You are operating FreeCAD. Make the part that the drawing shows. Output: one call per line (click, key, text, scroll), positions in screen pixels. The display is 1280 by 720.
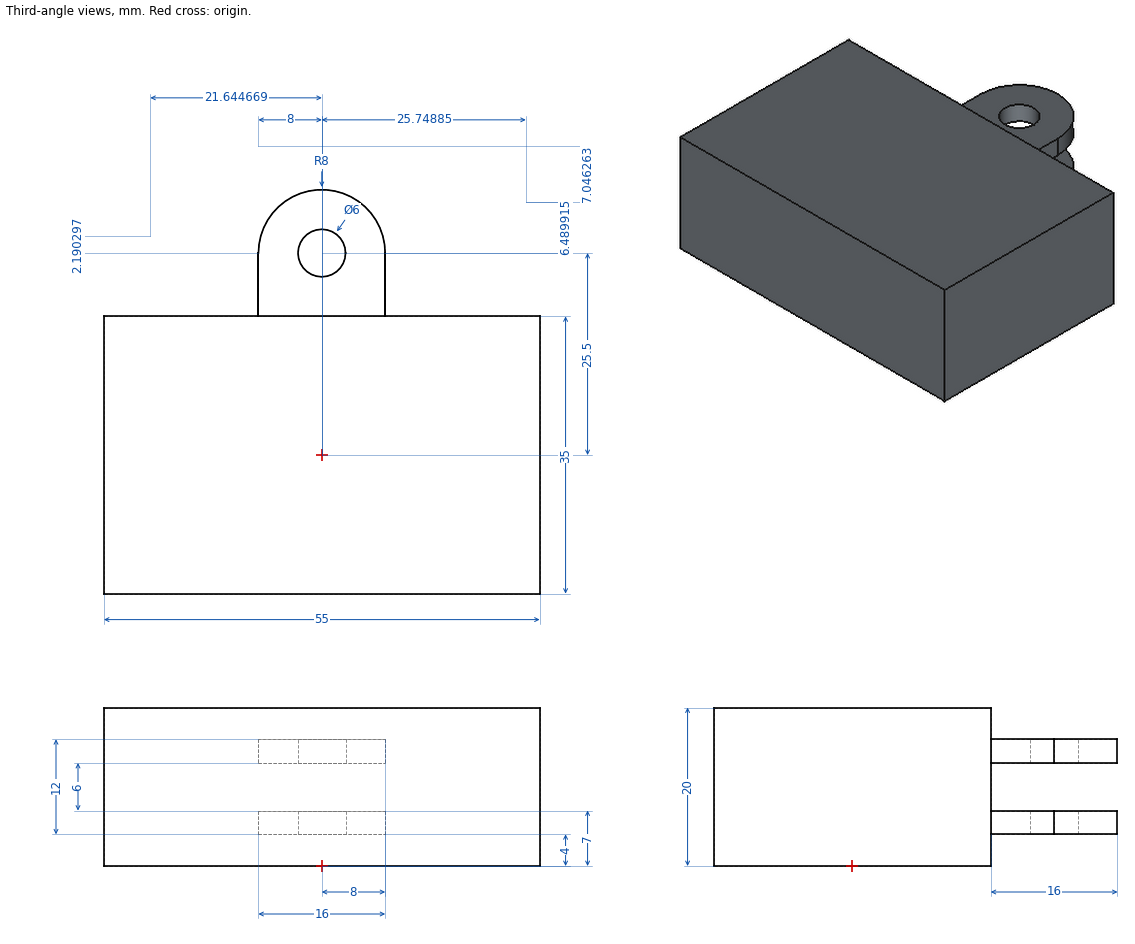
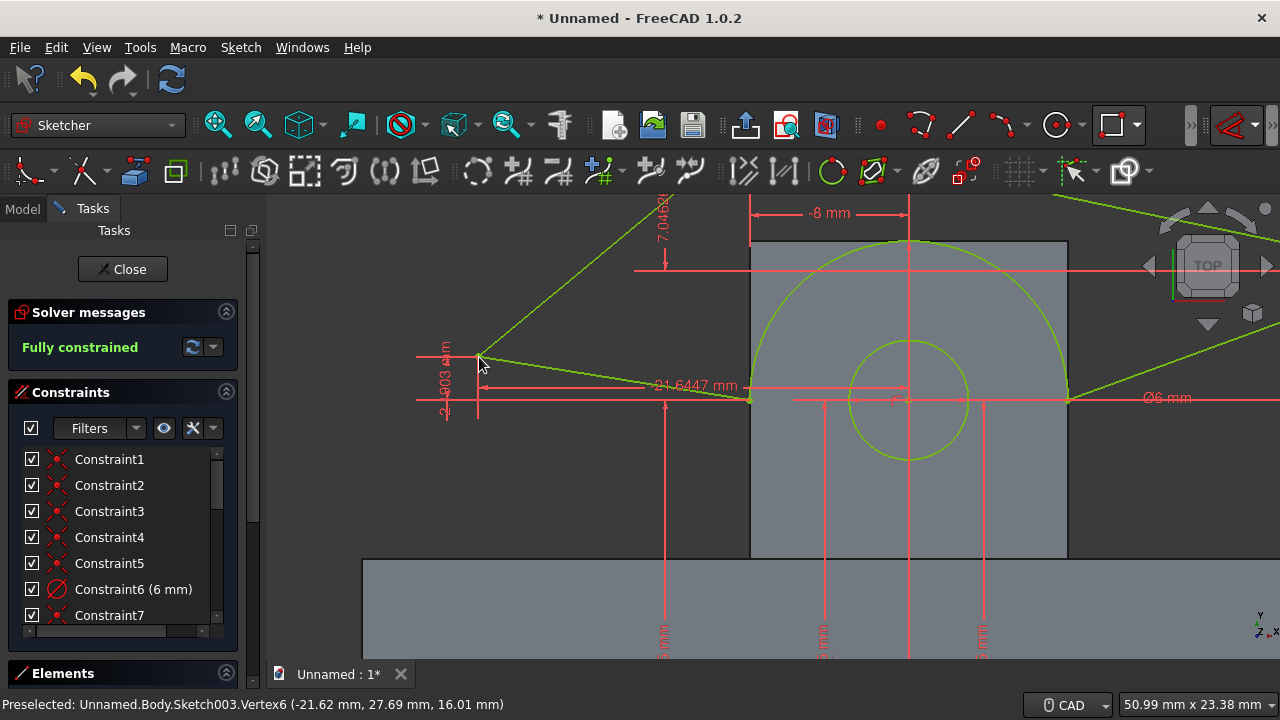
click(123, 269)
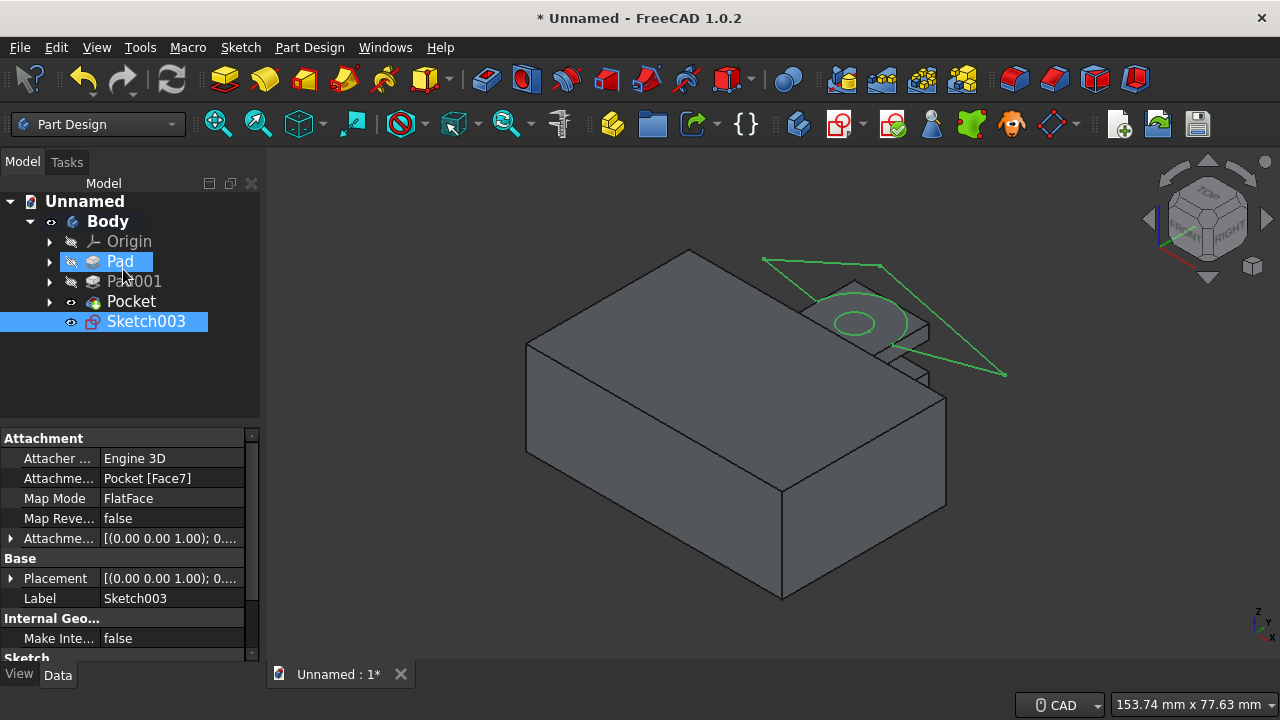
click(488, 80)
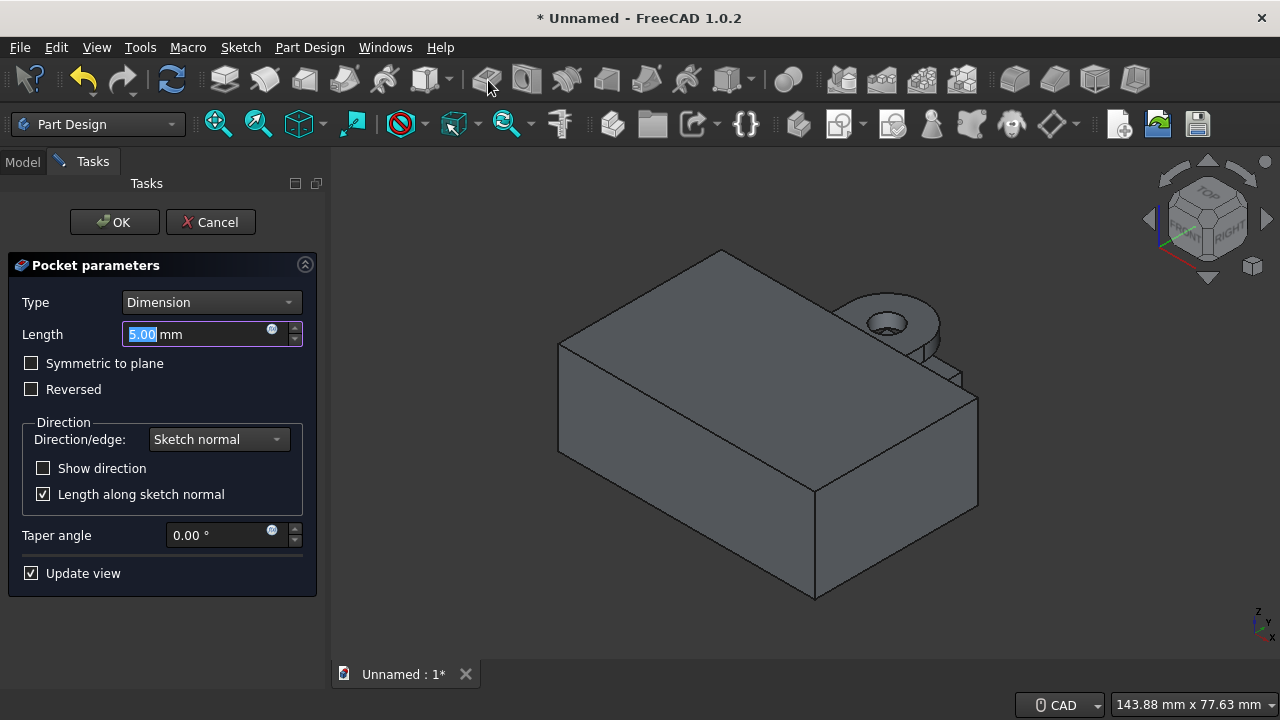
click(212, 302)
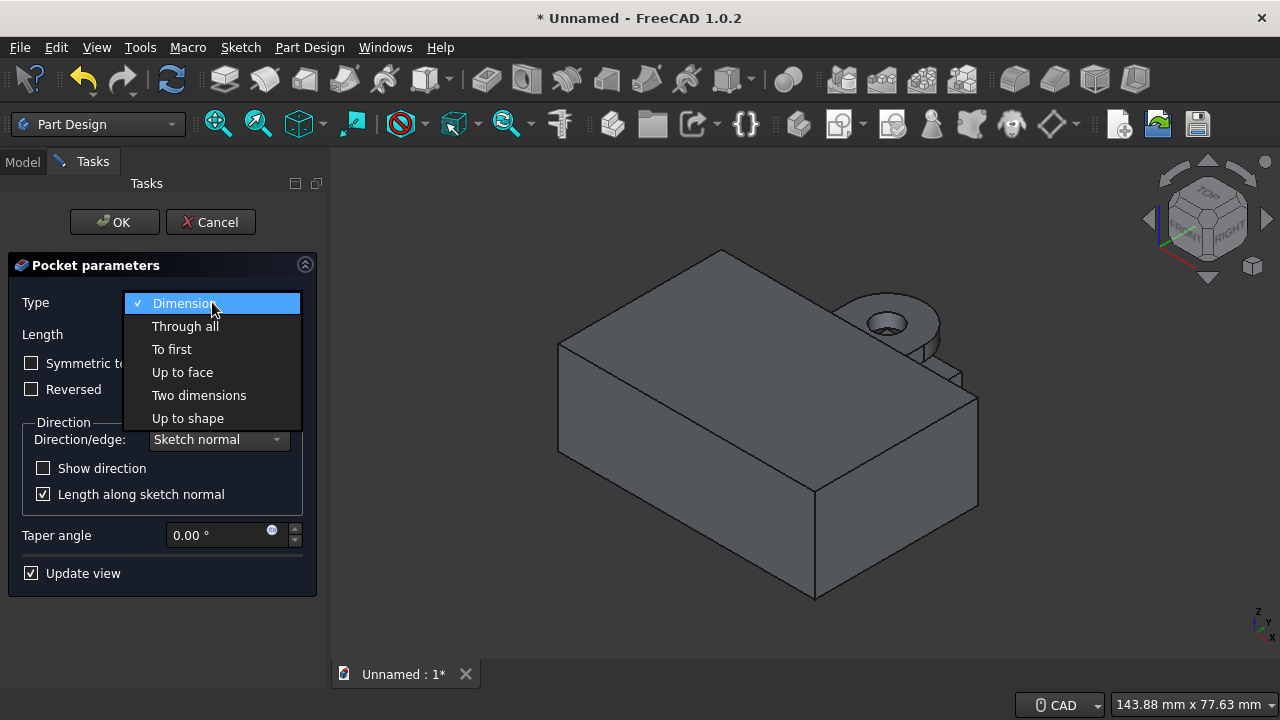
click(212, 326)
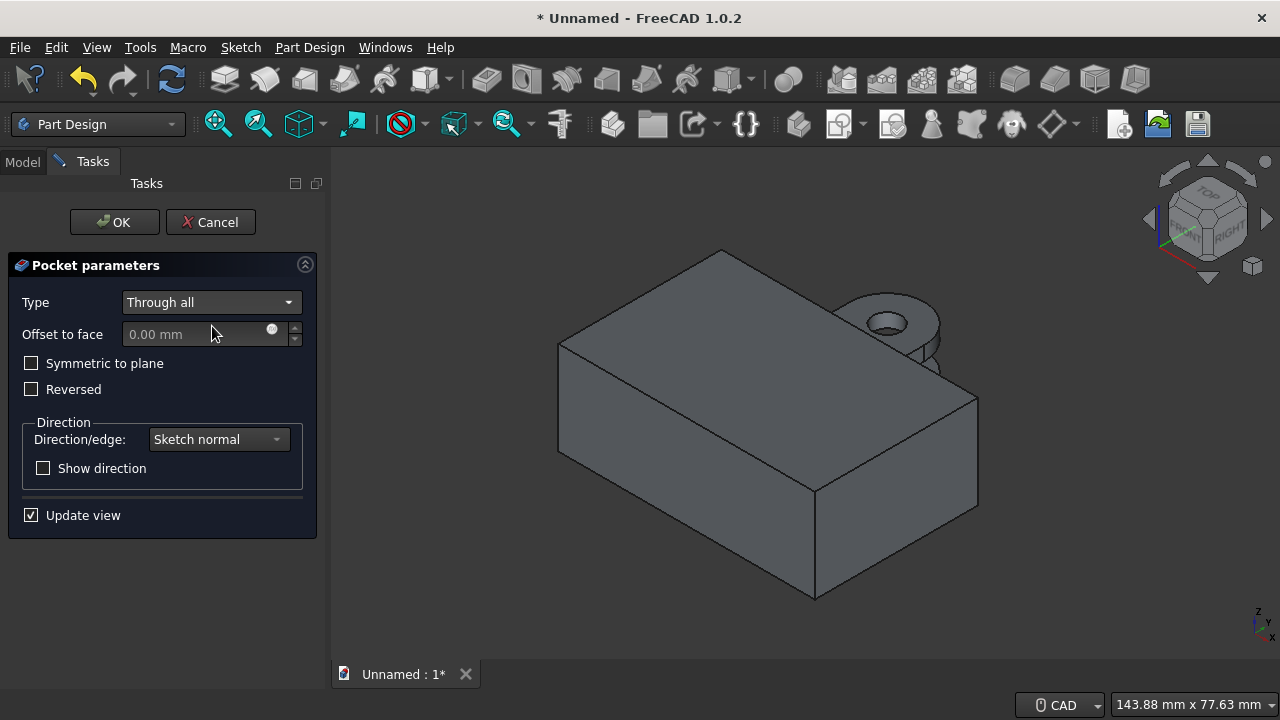
click(115, 222)